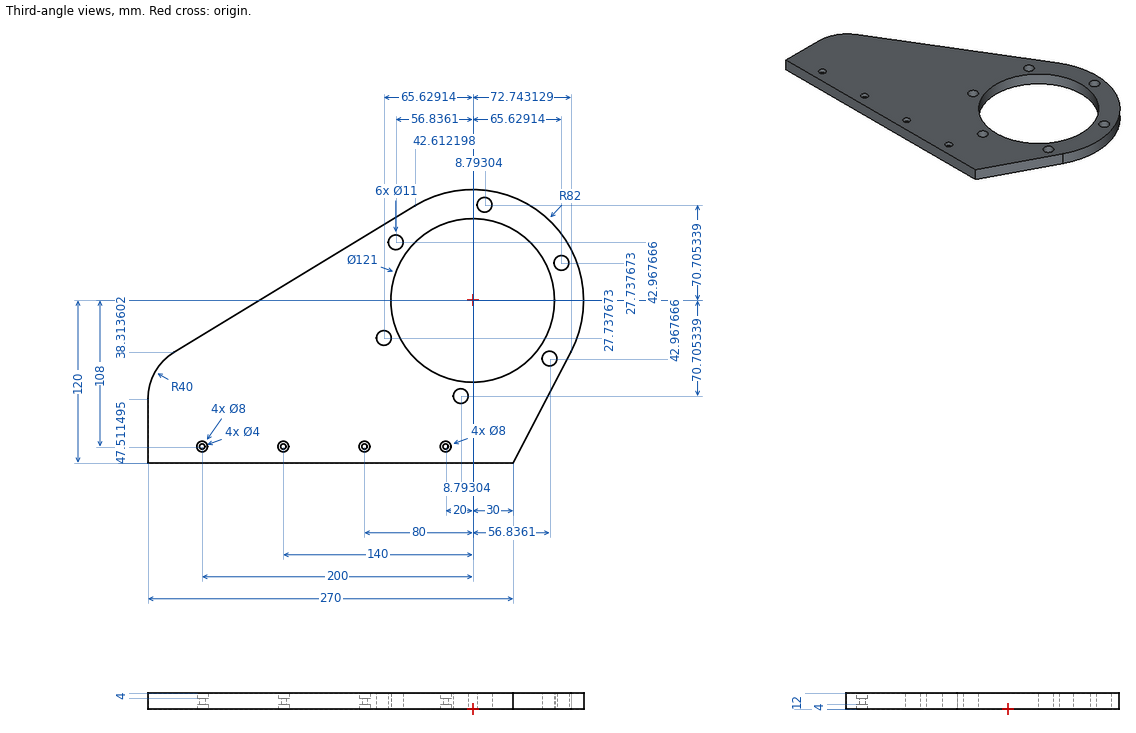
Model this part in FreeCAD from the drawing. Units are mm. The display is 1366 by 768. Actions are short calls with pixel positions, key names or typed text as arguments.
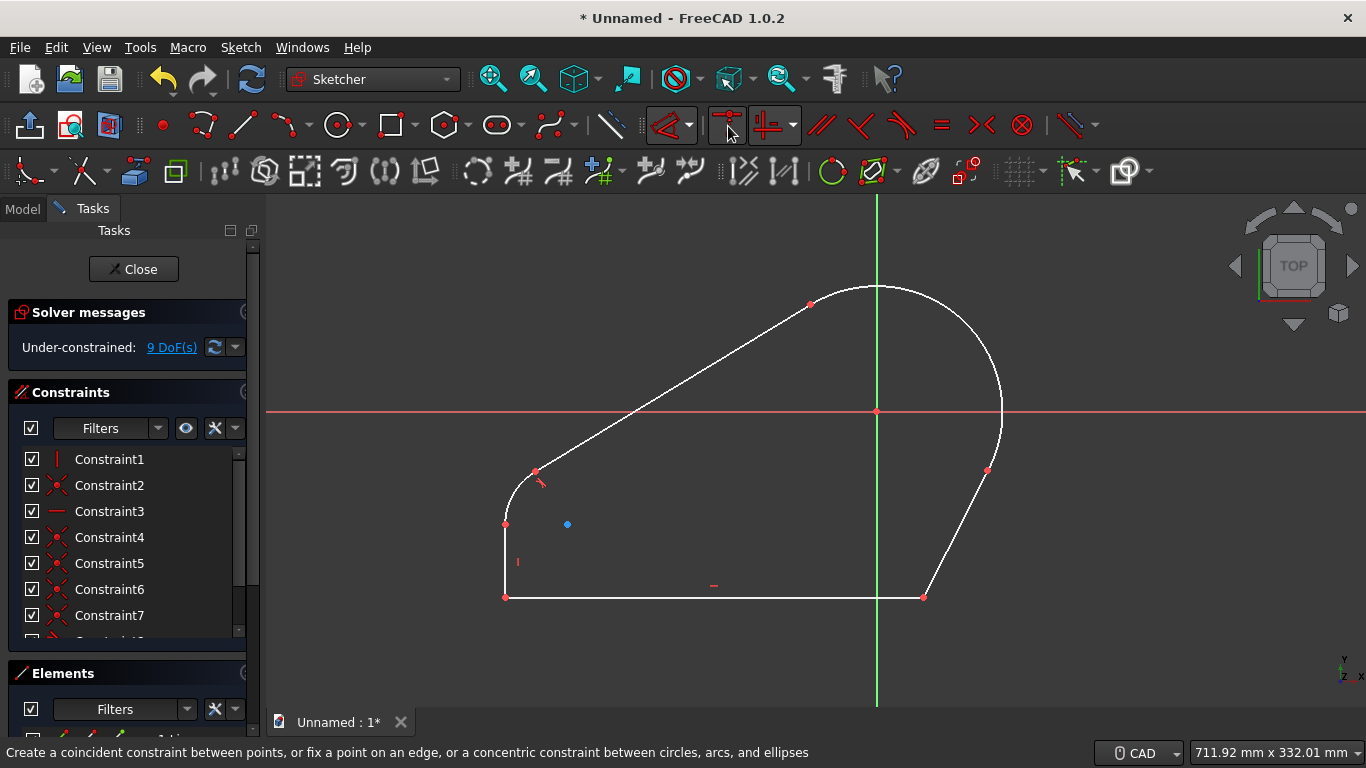
click(666, 126)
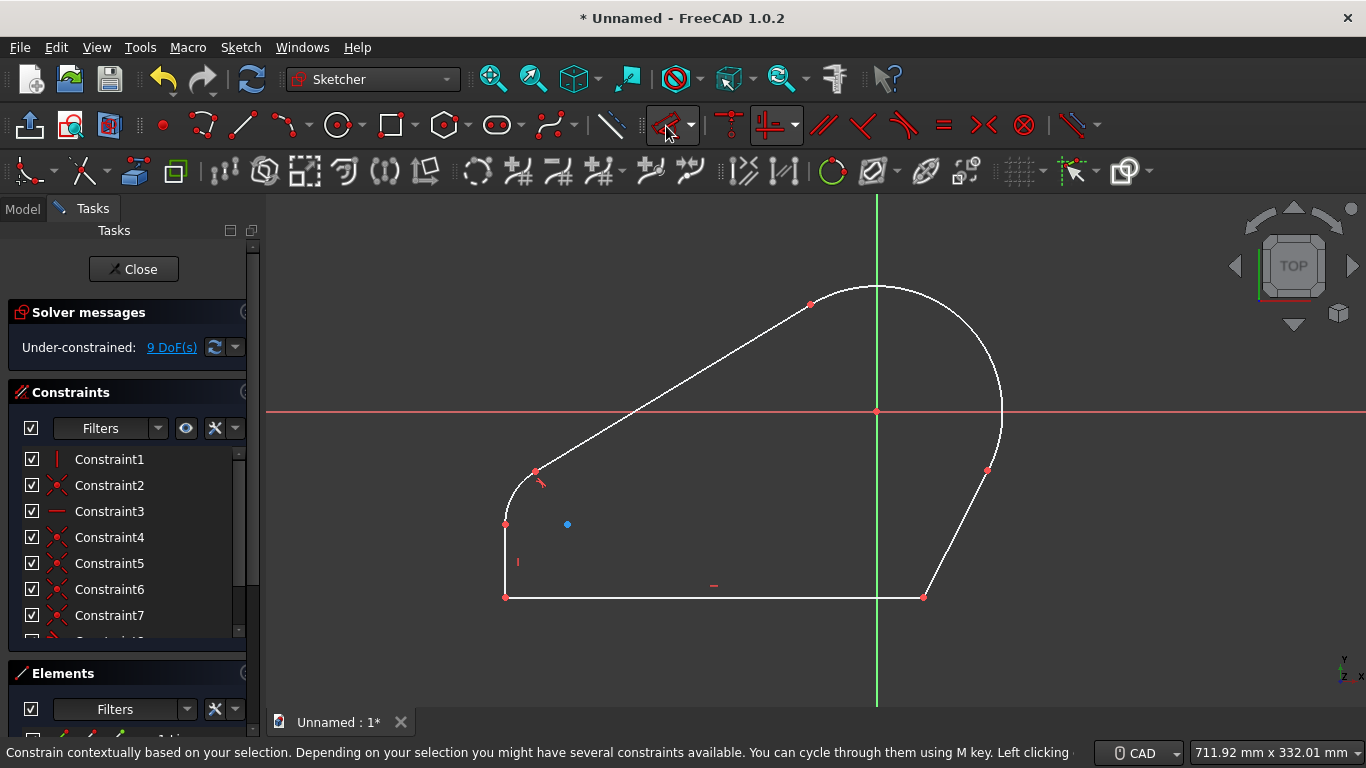
click(997, 375)
click(1028, 366)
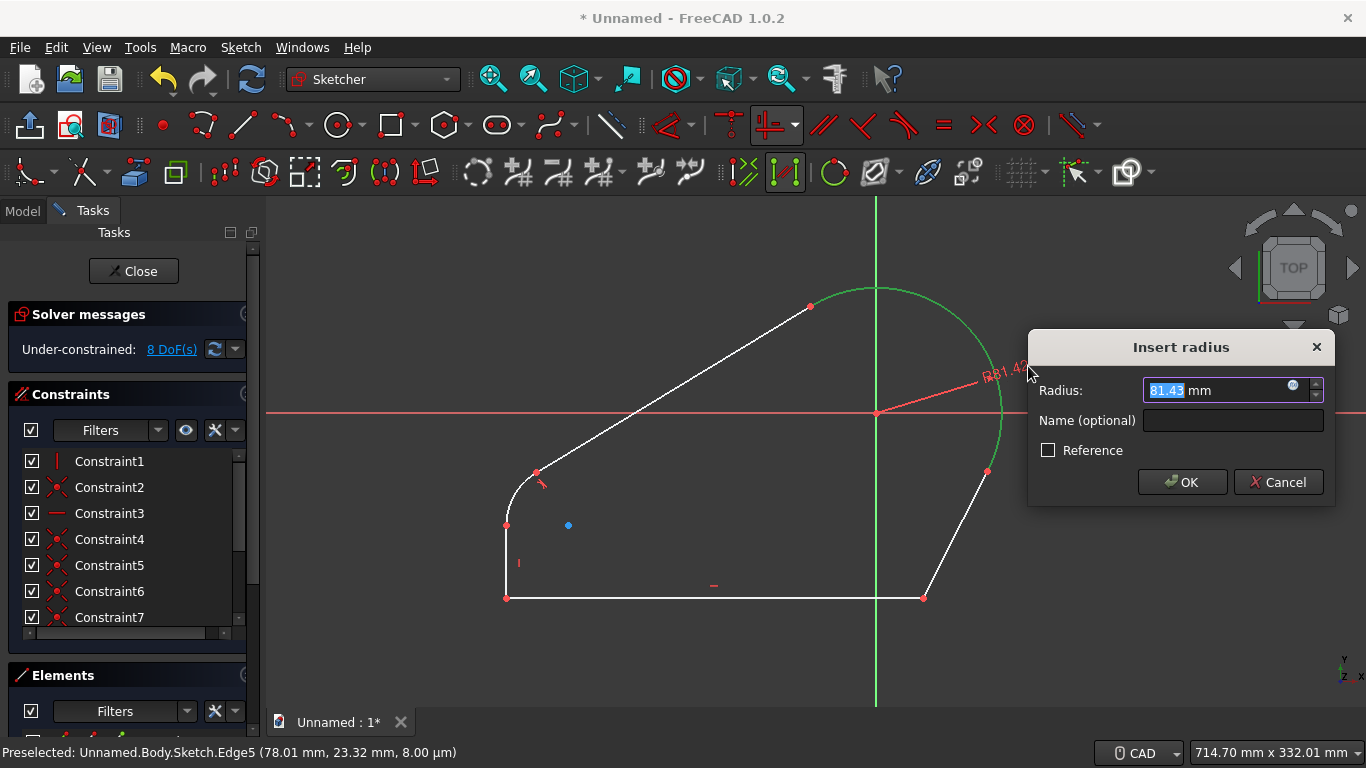
text(82)
key(Return)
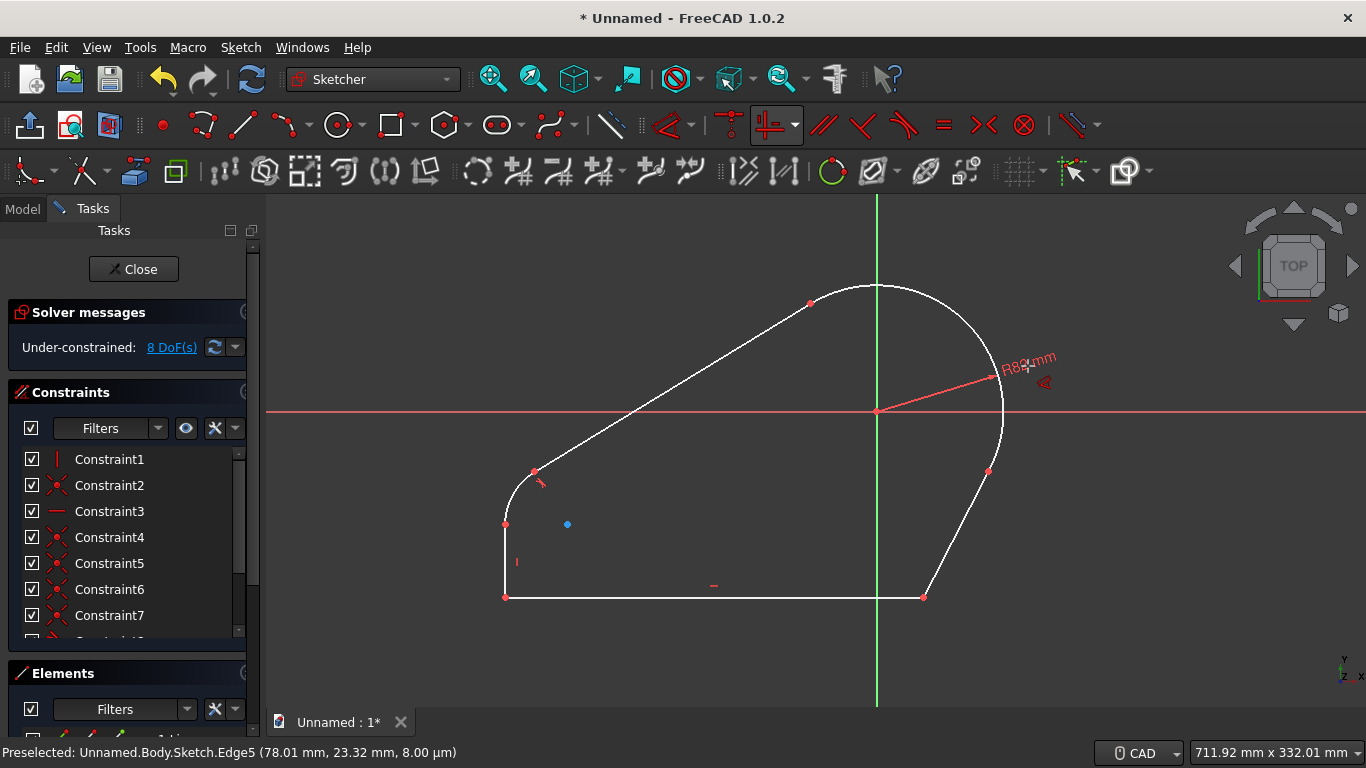
click(520, 484)
click(496, 463)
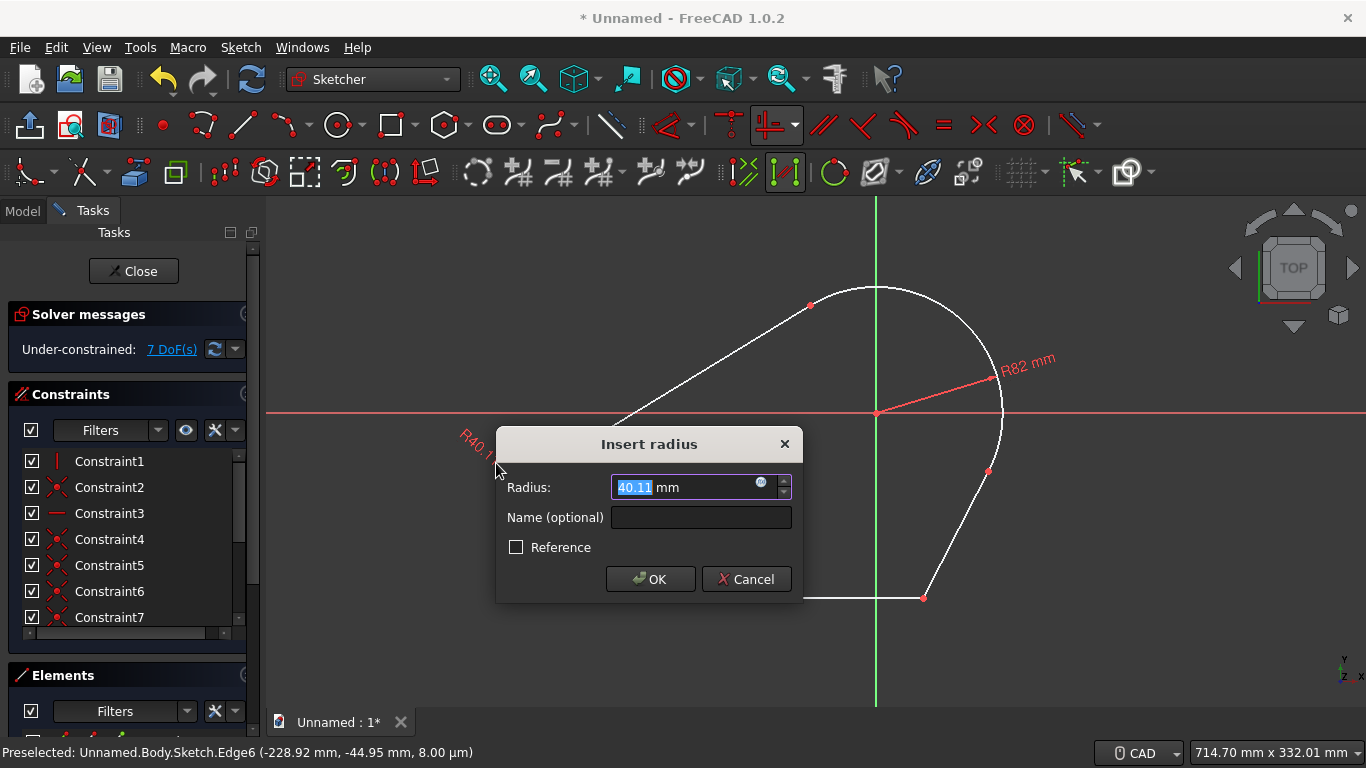
text(40)
key(Return)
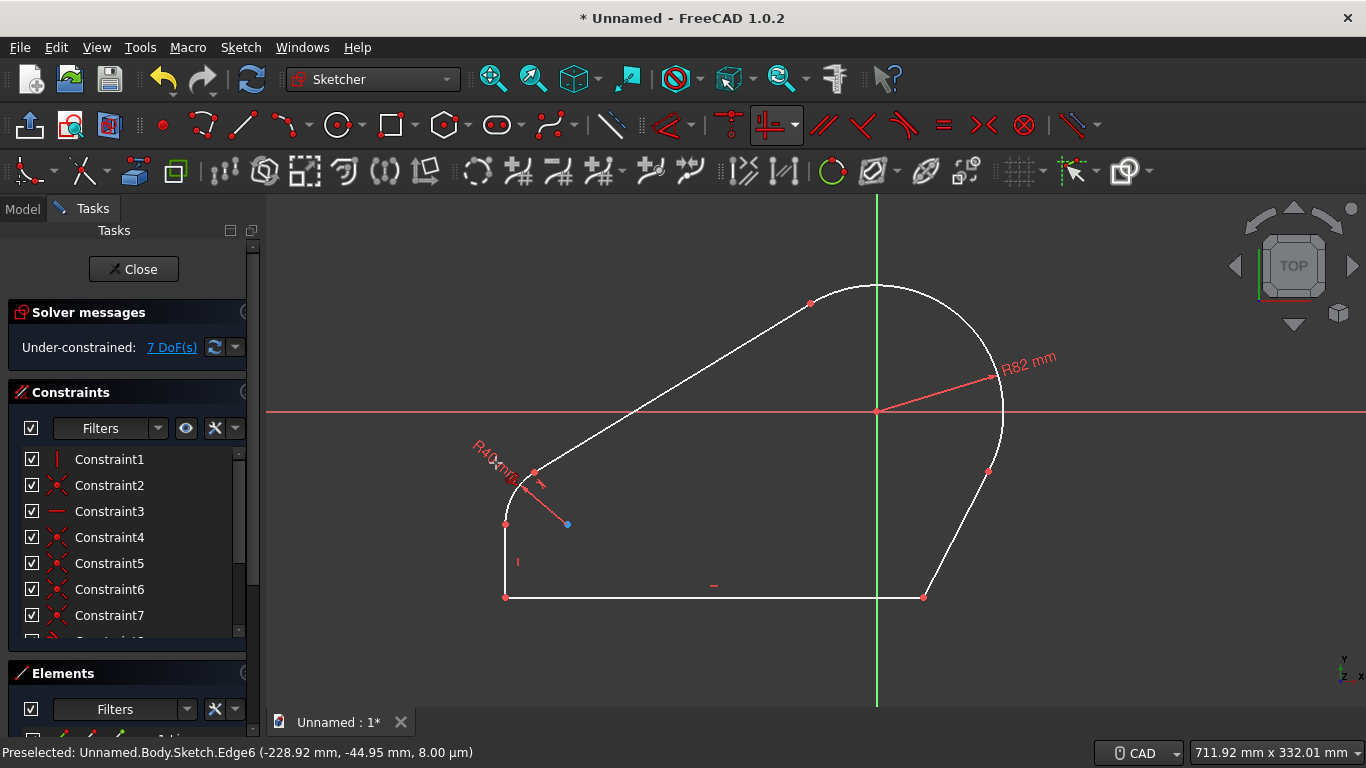
click(631, 598)
click(714, 632)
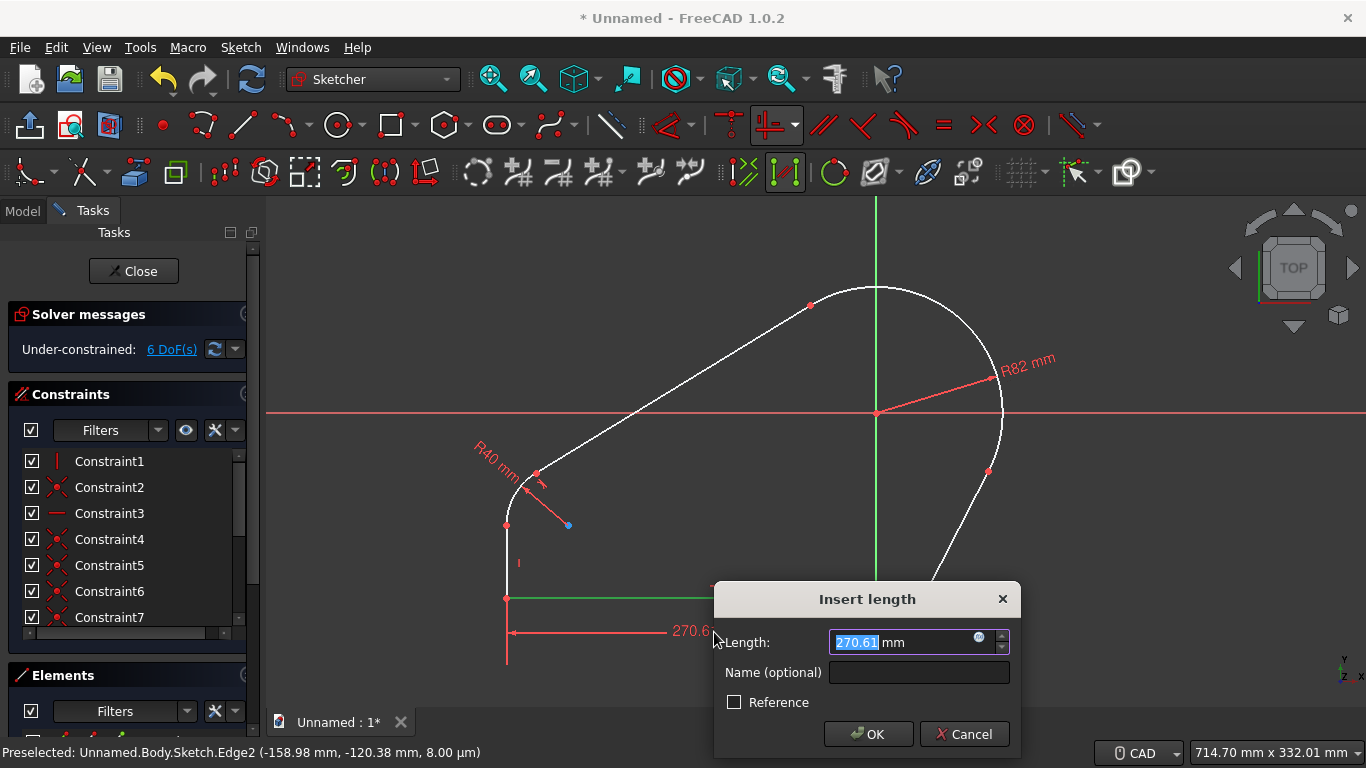
text(270)
key(Return)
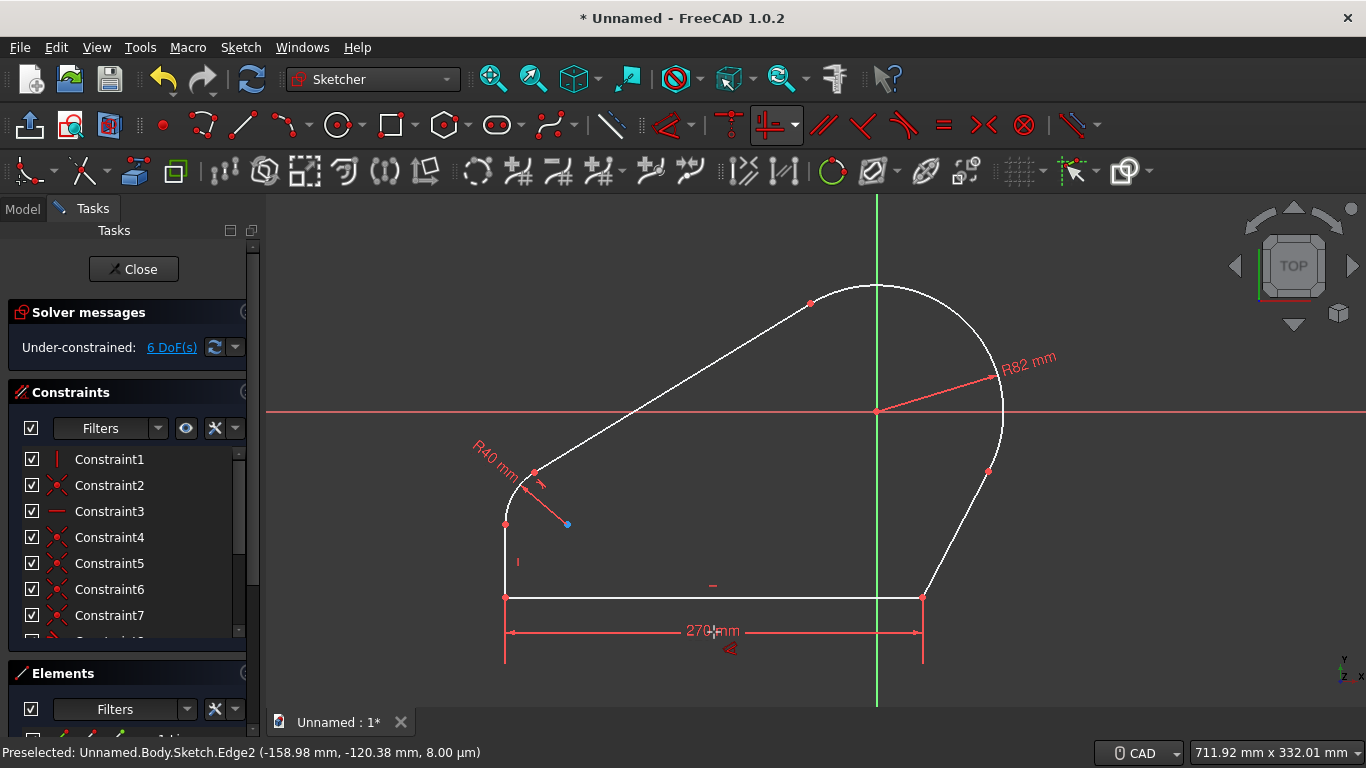
click(923, 598)
click(900, 632)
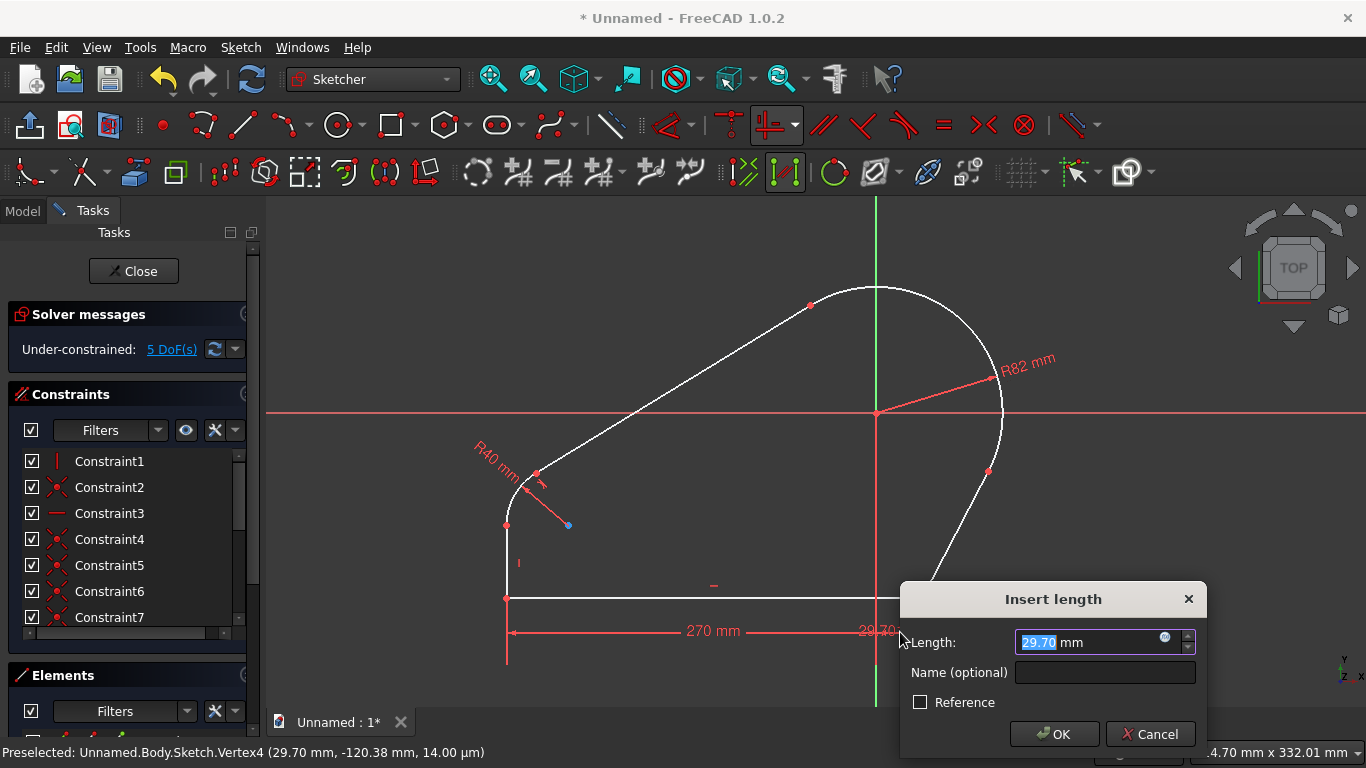
text(30)
key(Return)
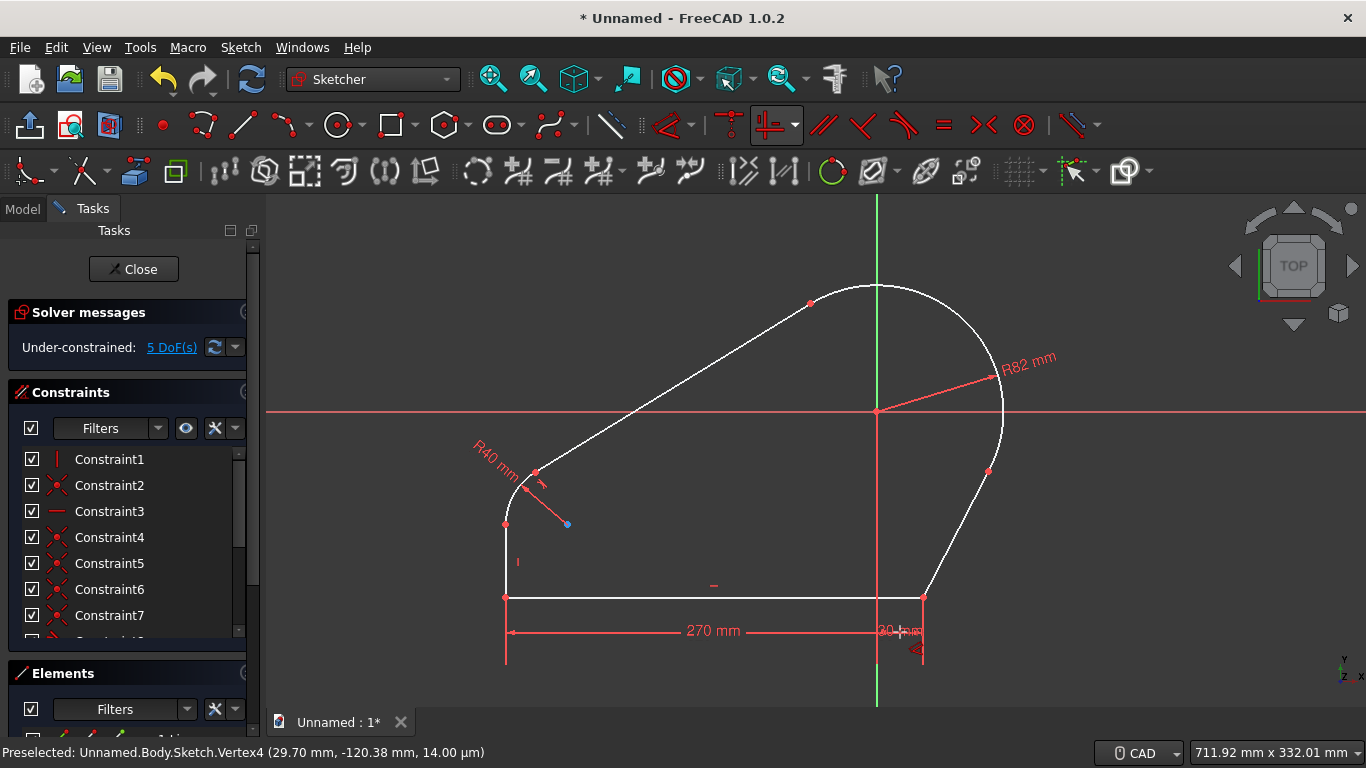
click(506, 598)
click(472, 505)